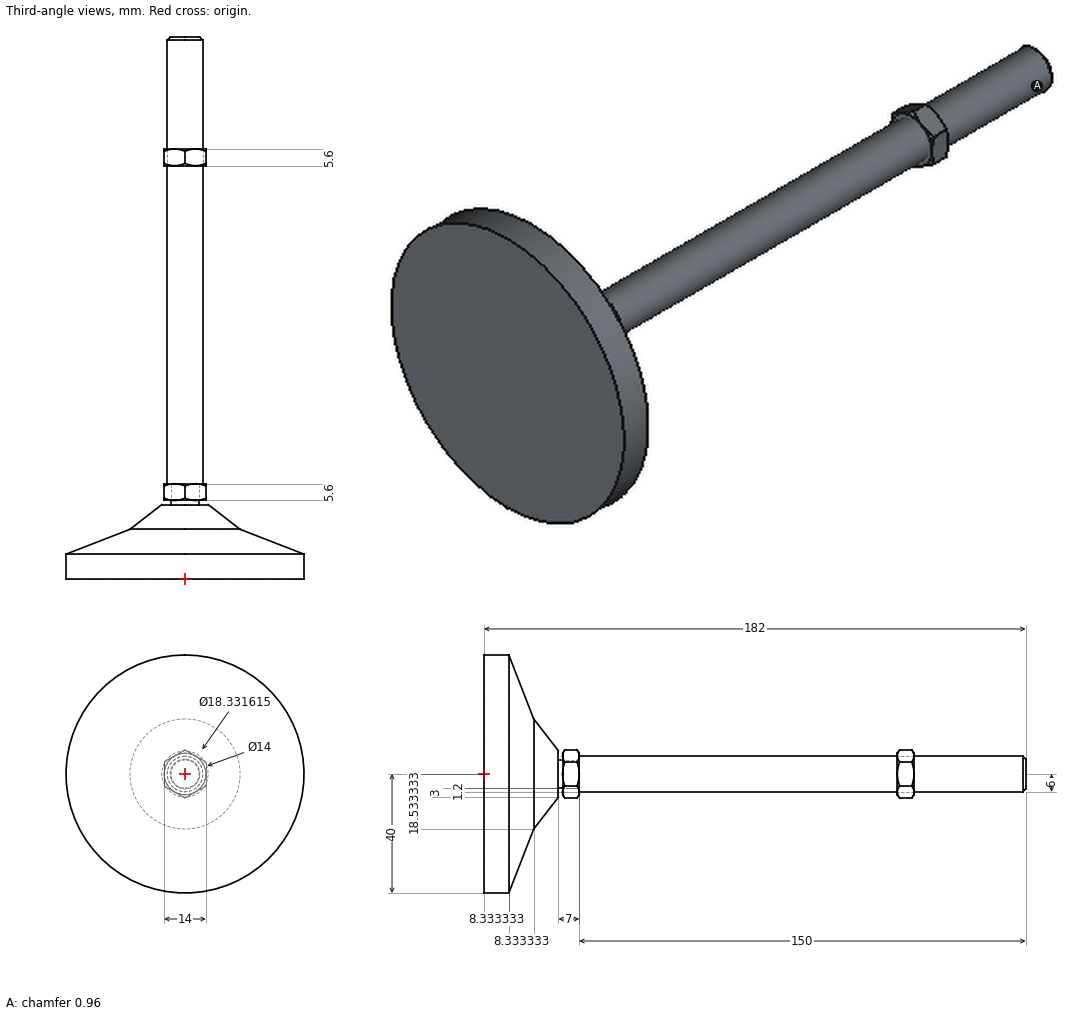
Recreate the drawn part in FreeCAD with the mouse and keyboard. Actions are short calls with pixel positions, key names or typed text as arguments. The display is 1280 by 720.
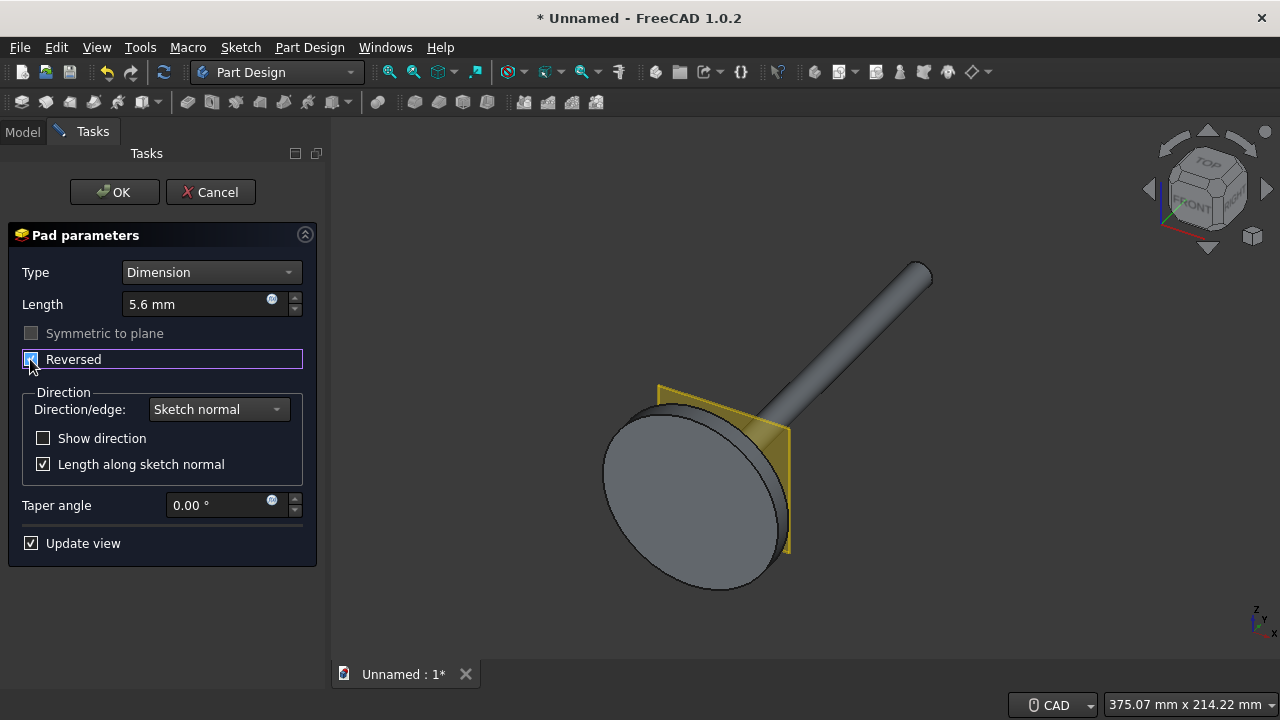
click(115, 192)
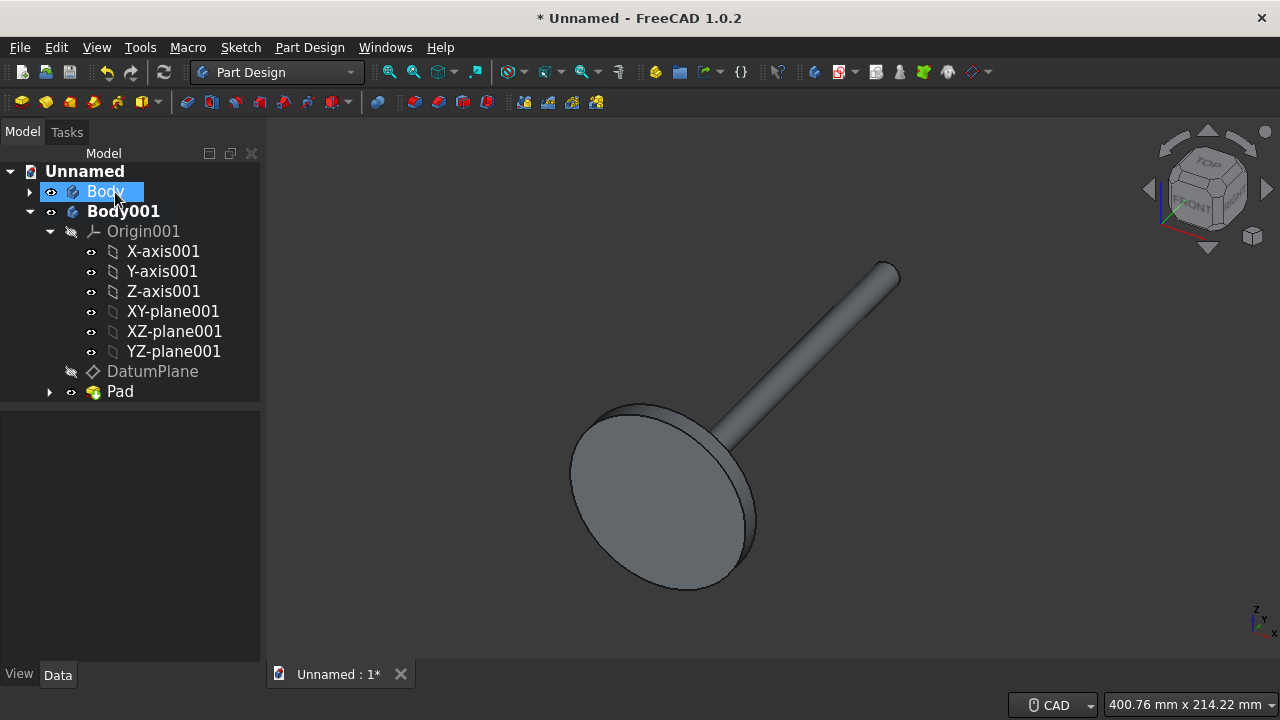
click(390, 72)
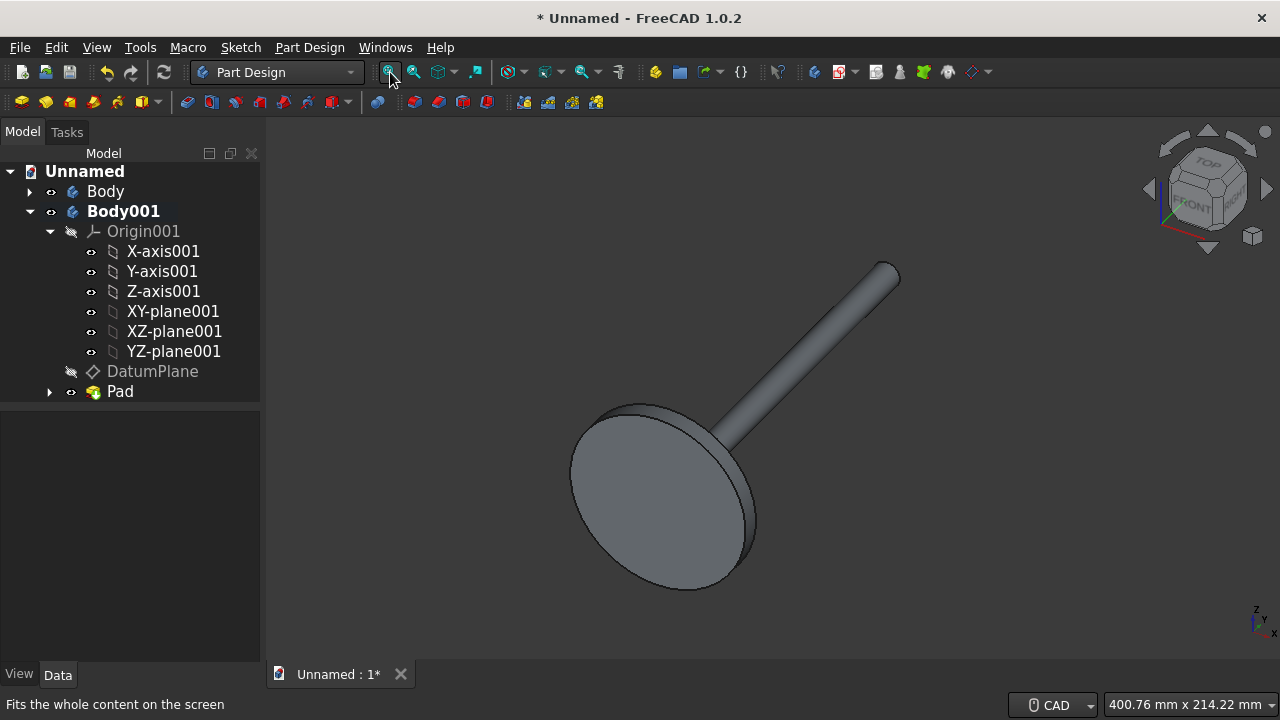
key(4)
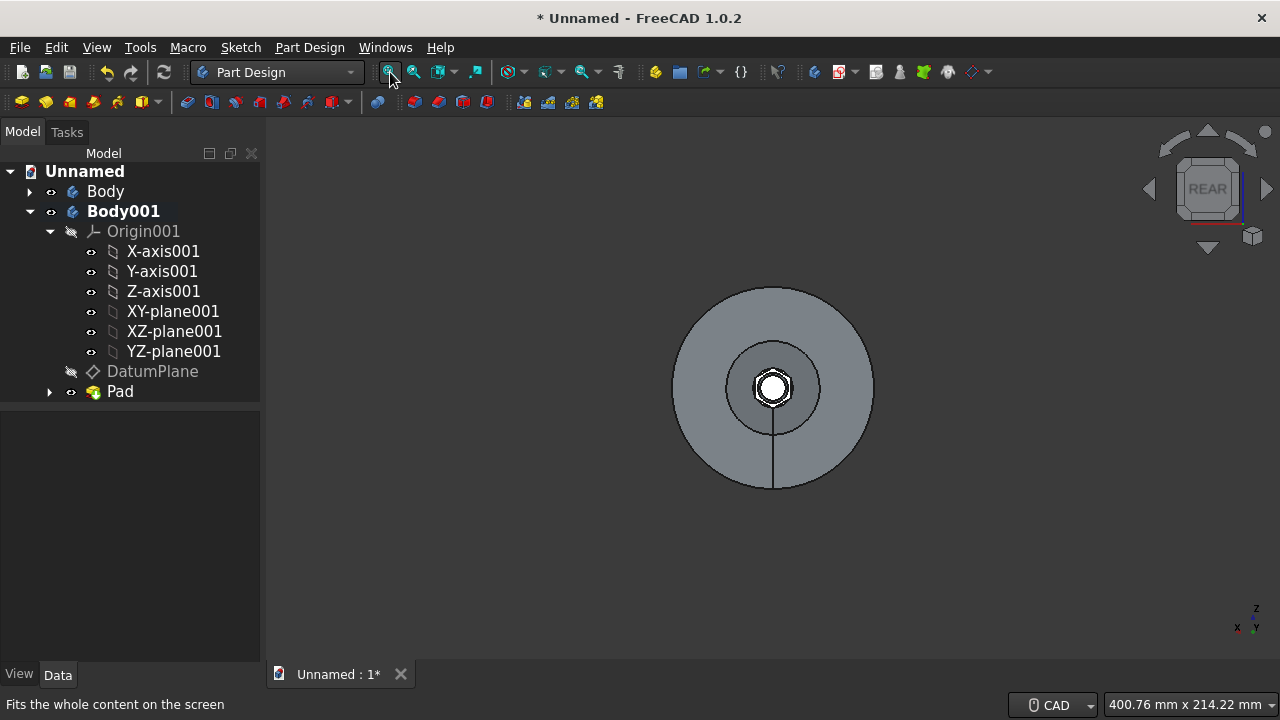
click(390, 72)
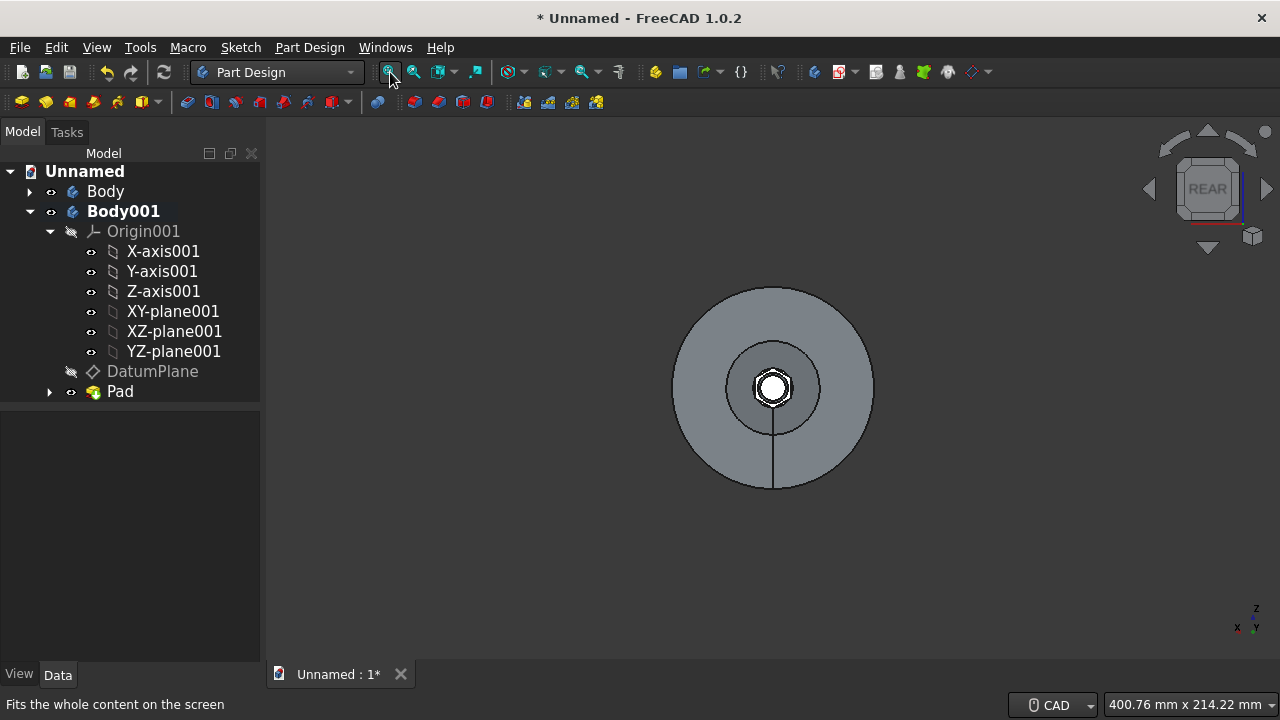
key(5)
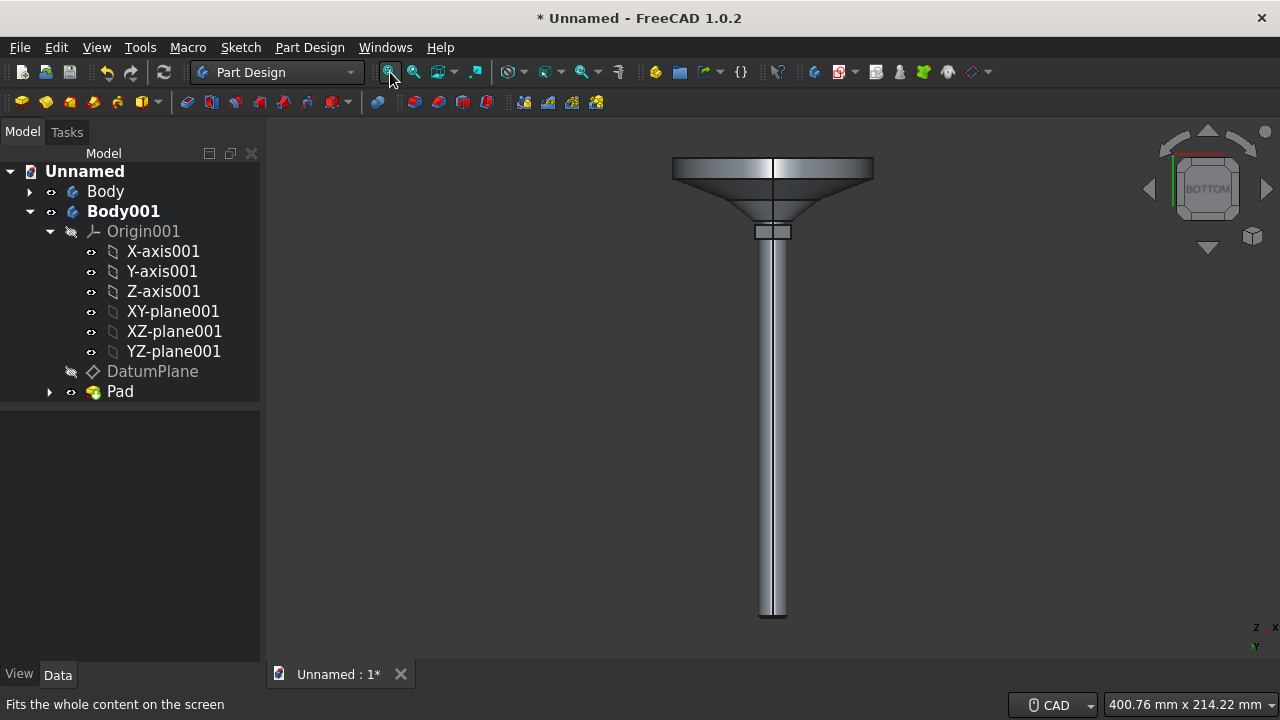
click(390, 72)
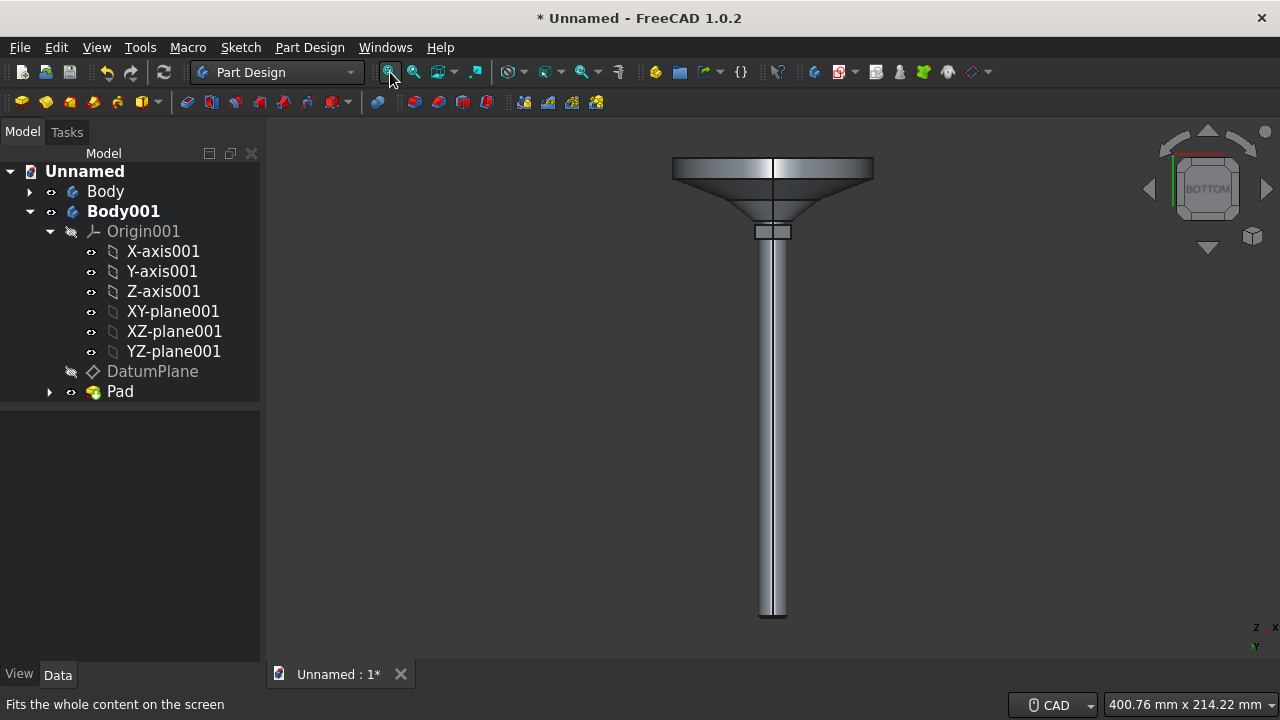
key(3)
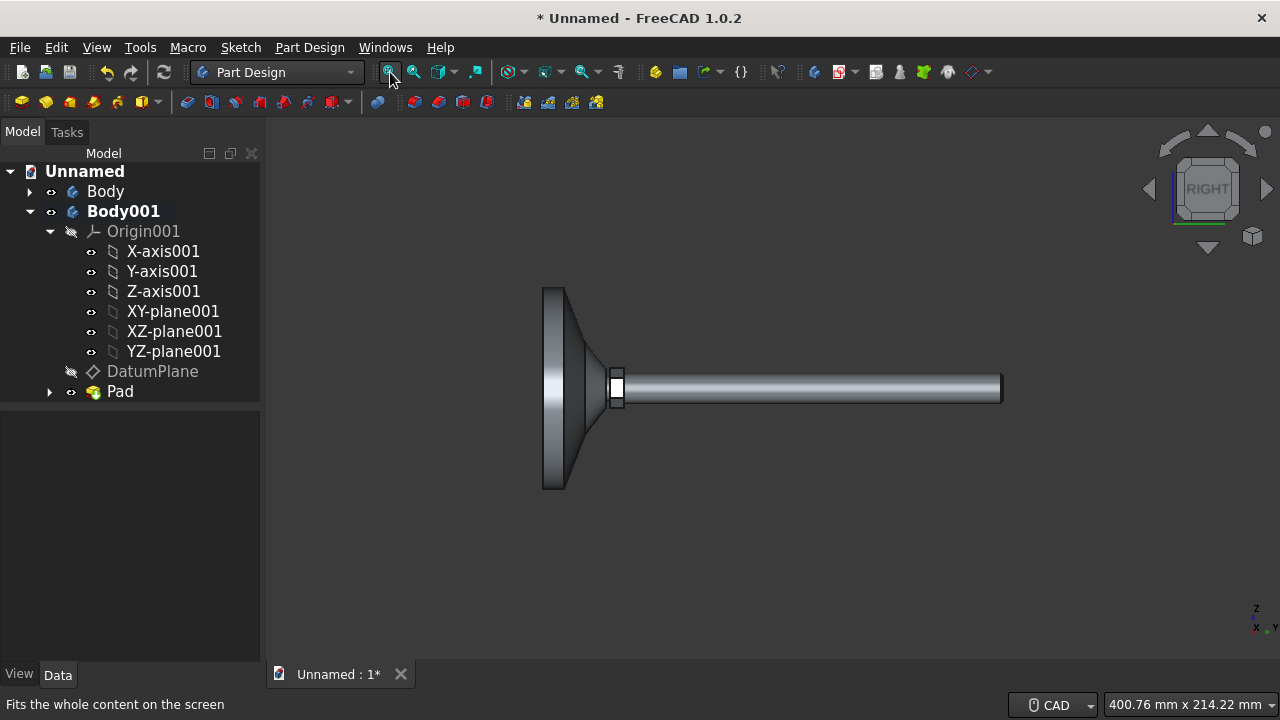
click(390, 72)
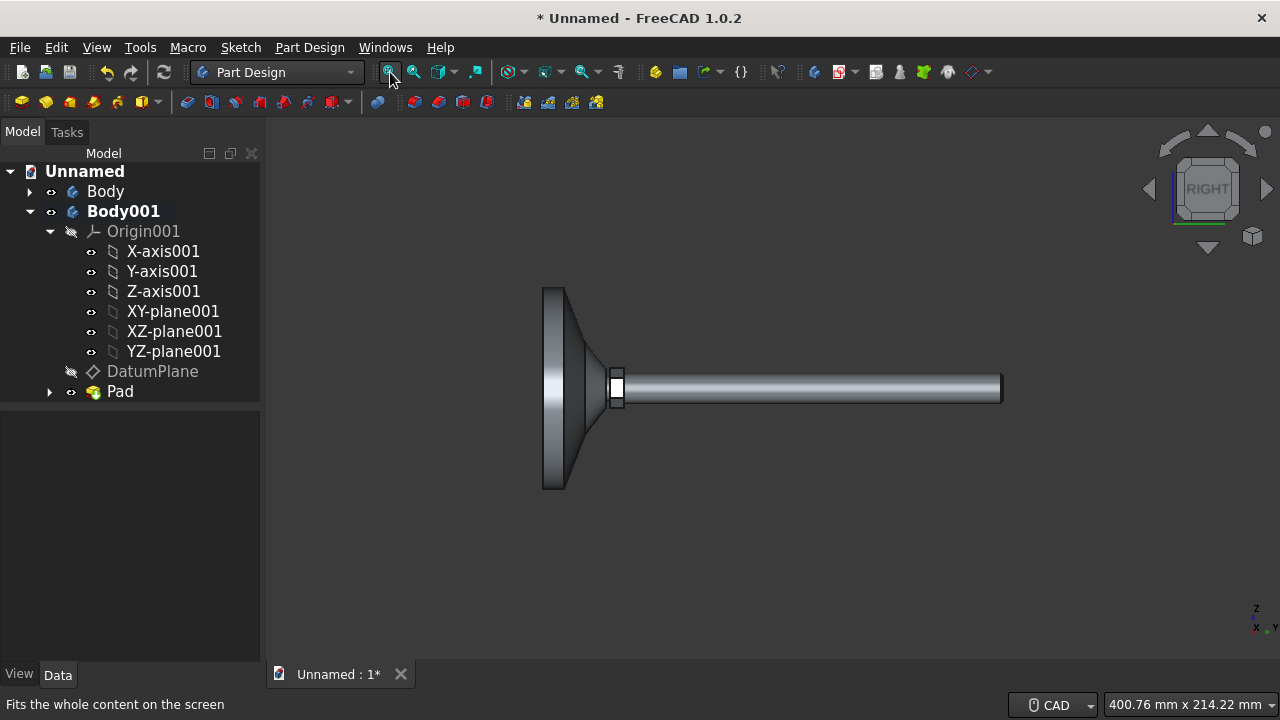
click(136, 332)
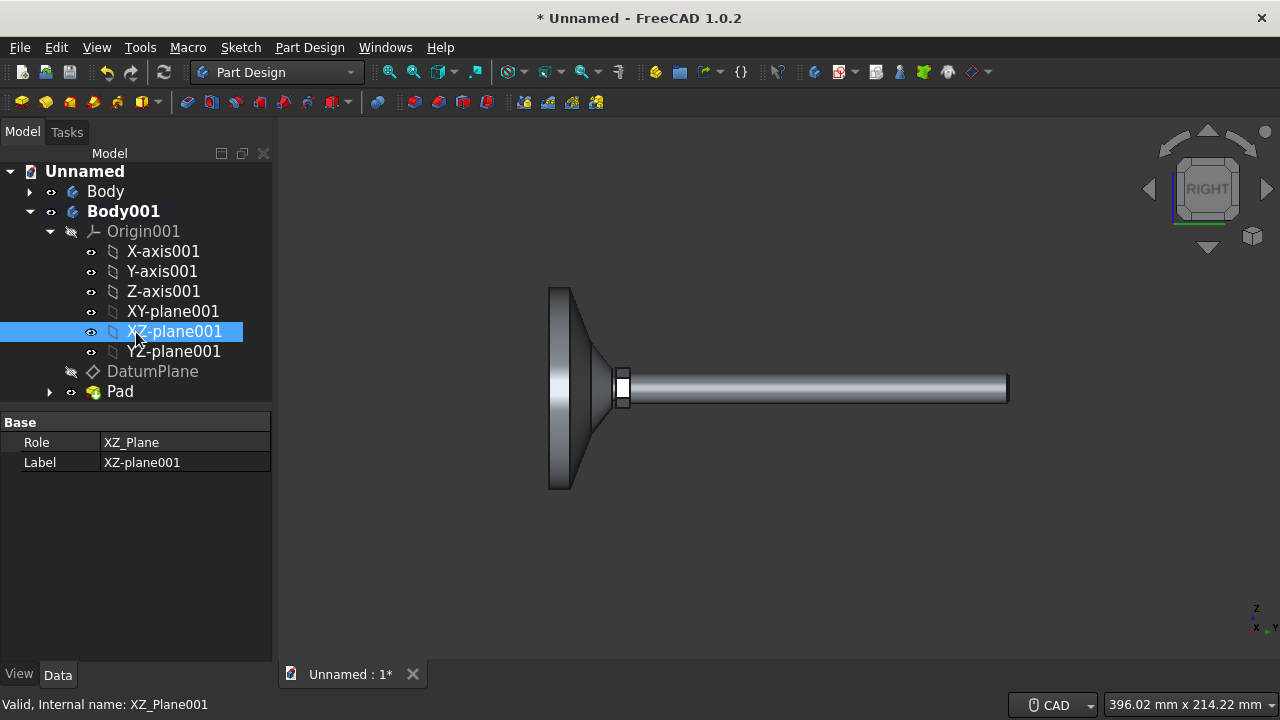
click(972, 72)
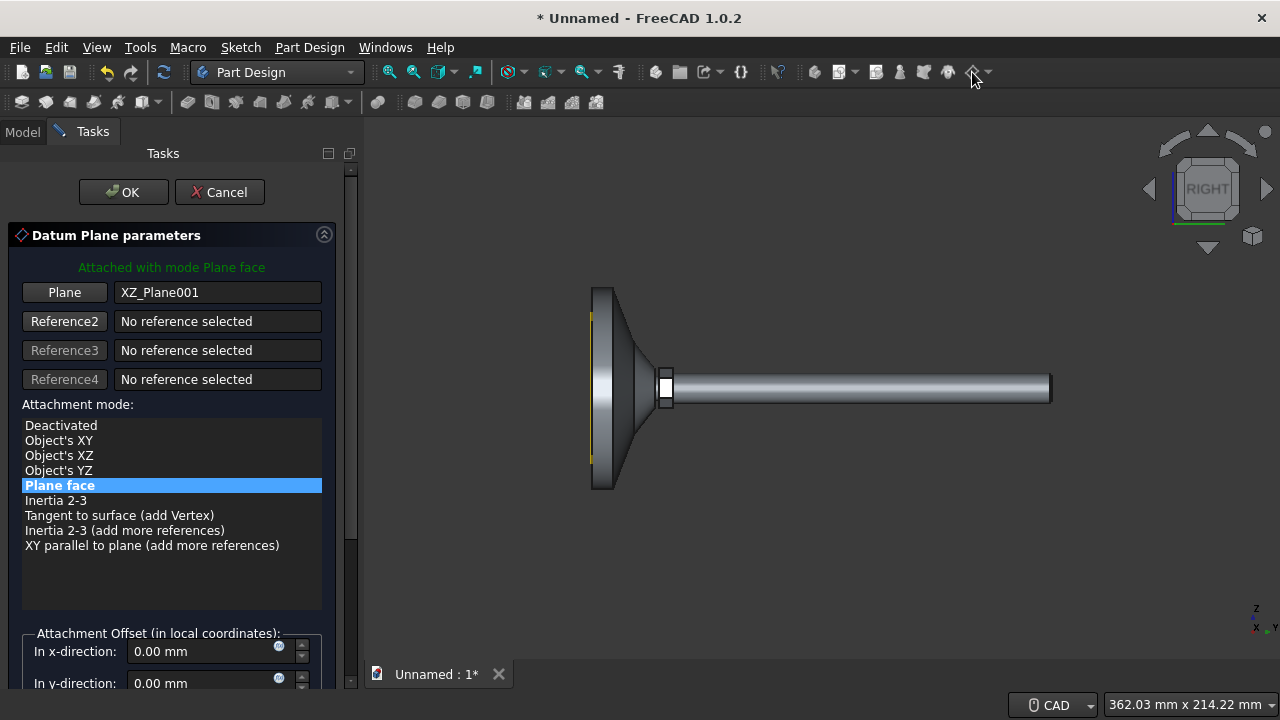
scroll(351, 426, down, 2)